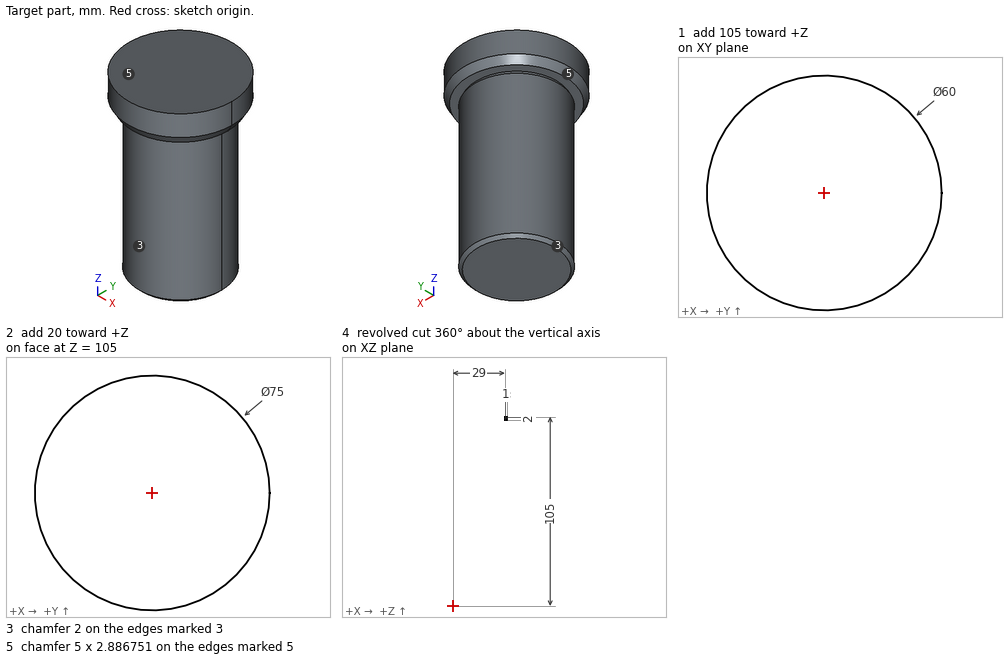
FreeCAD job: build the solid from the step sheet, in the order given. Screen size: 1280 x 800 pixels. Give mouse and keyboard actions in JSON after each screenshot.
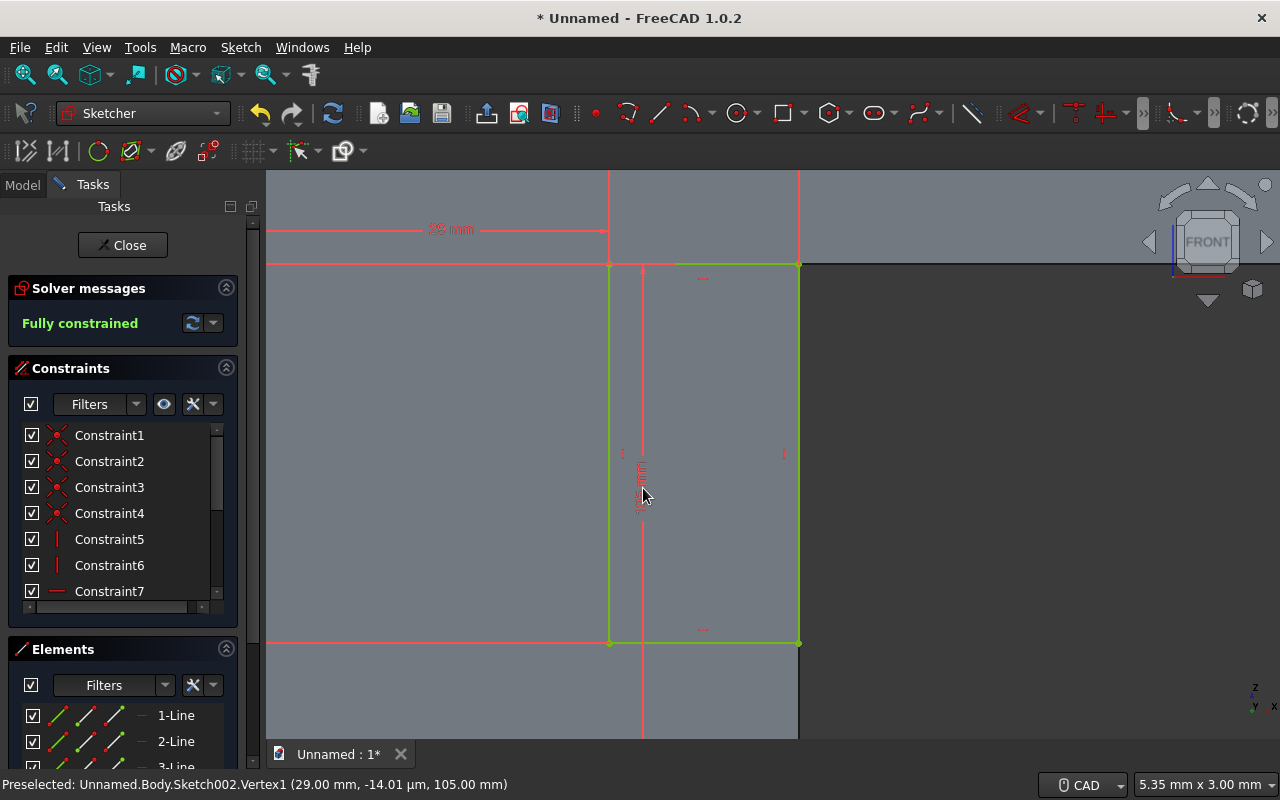
{"action": "left_click", "coordinate": [123, 245]}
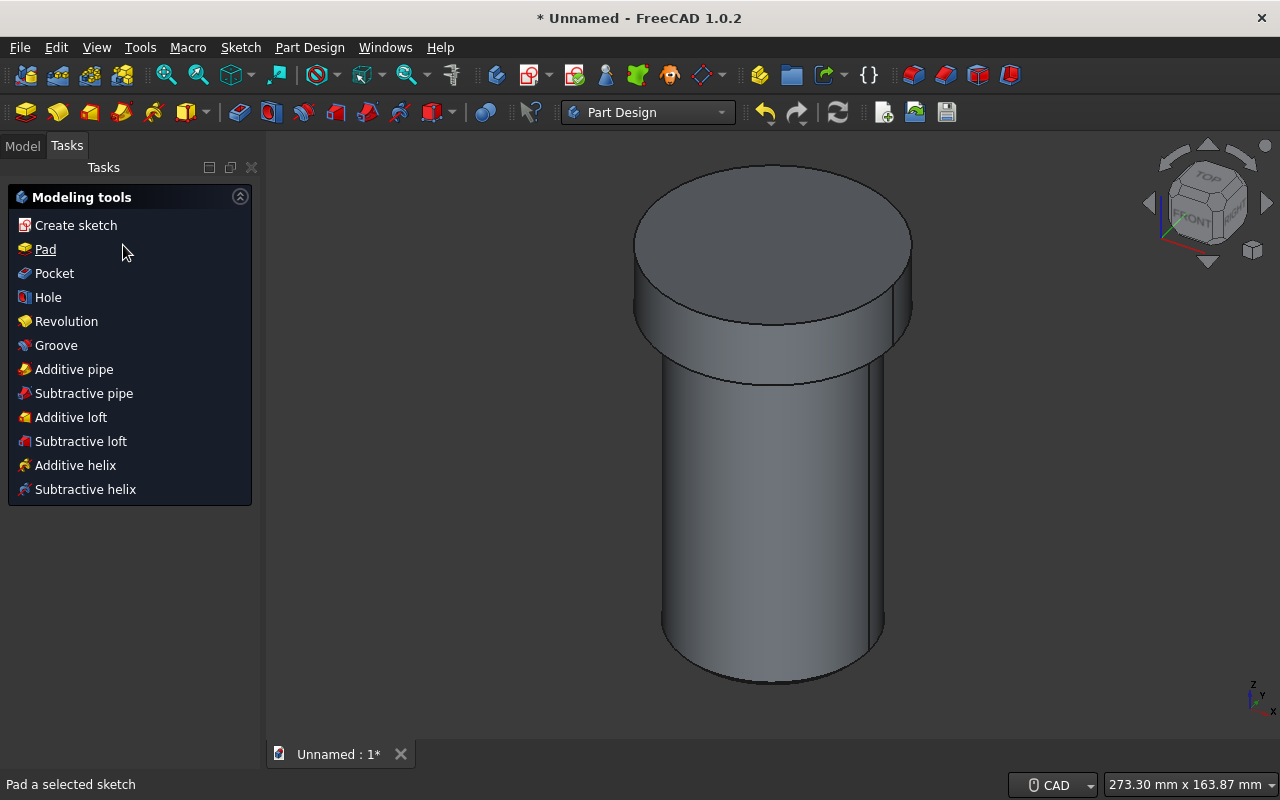
{"action": "left_click", "coordinate": [304, 112]}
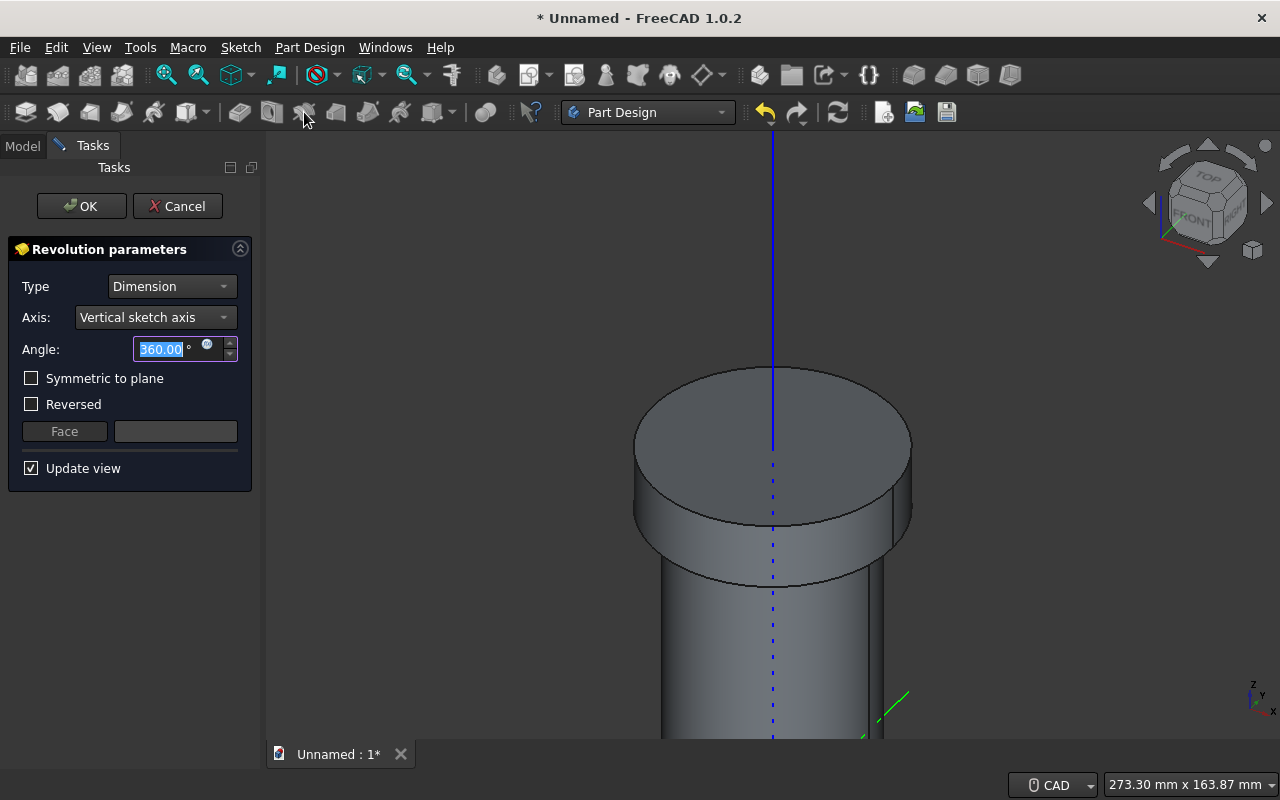
{"action": "left_click", "coordinate": [82, 206]}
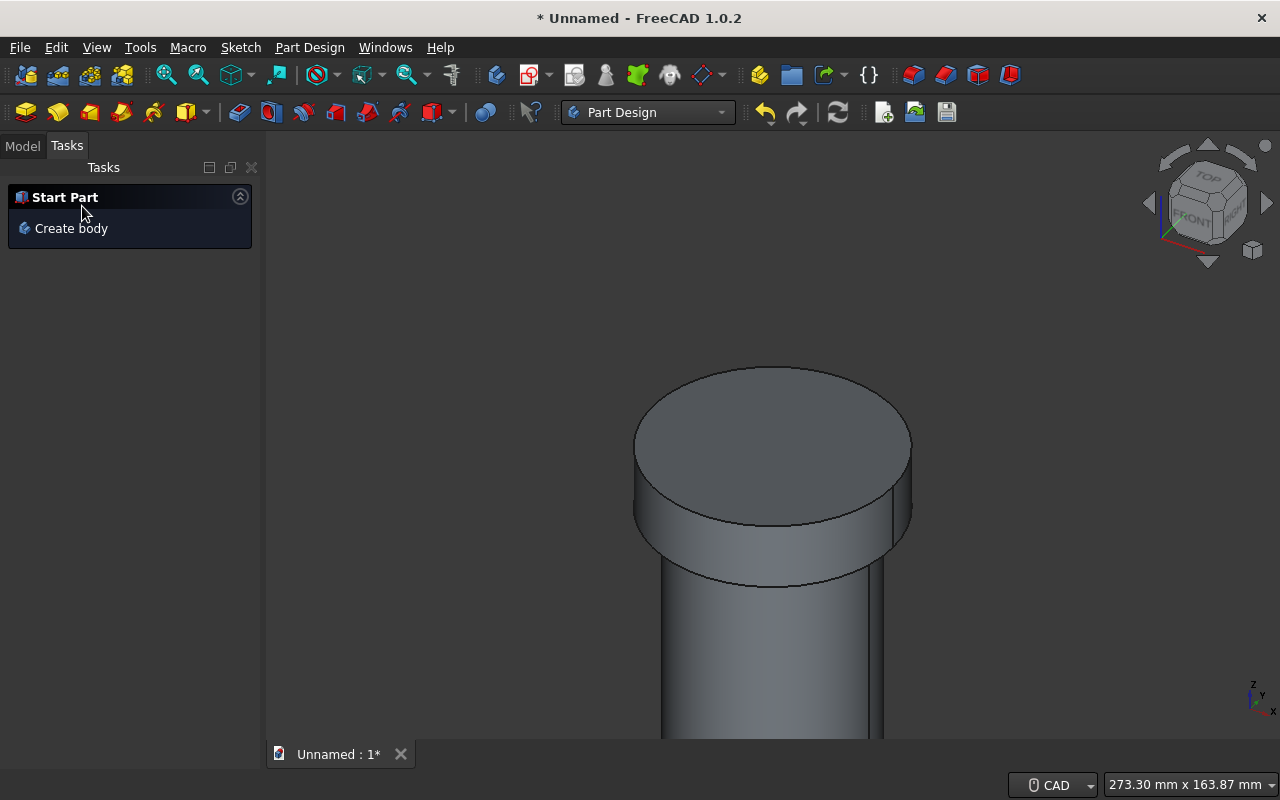
{"action": "left_click", "coordinate": [168, 76]}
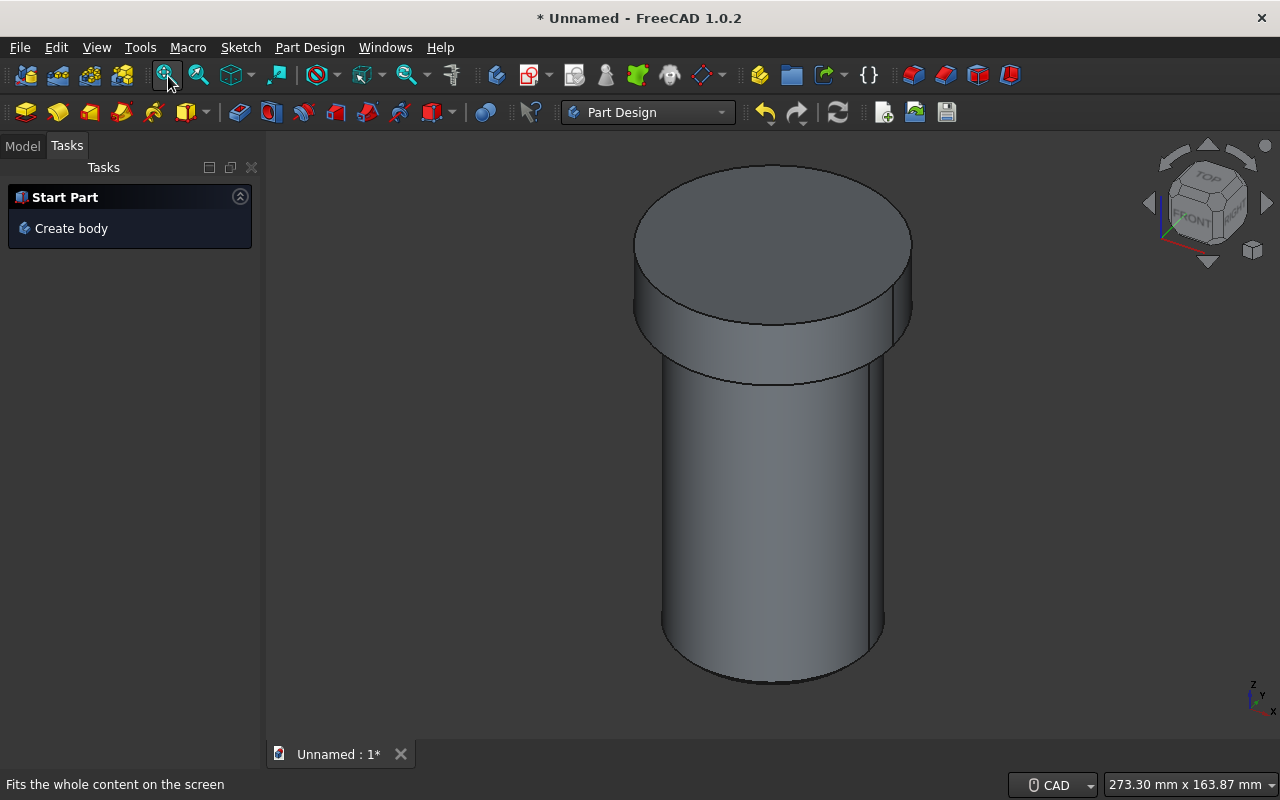
{"action": "key", "text": "0"}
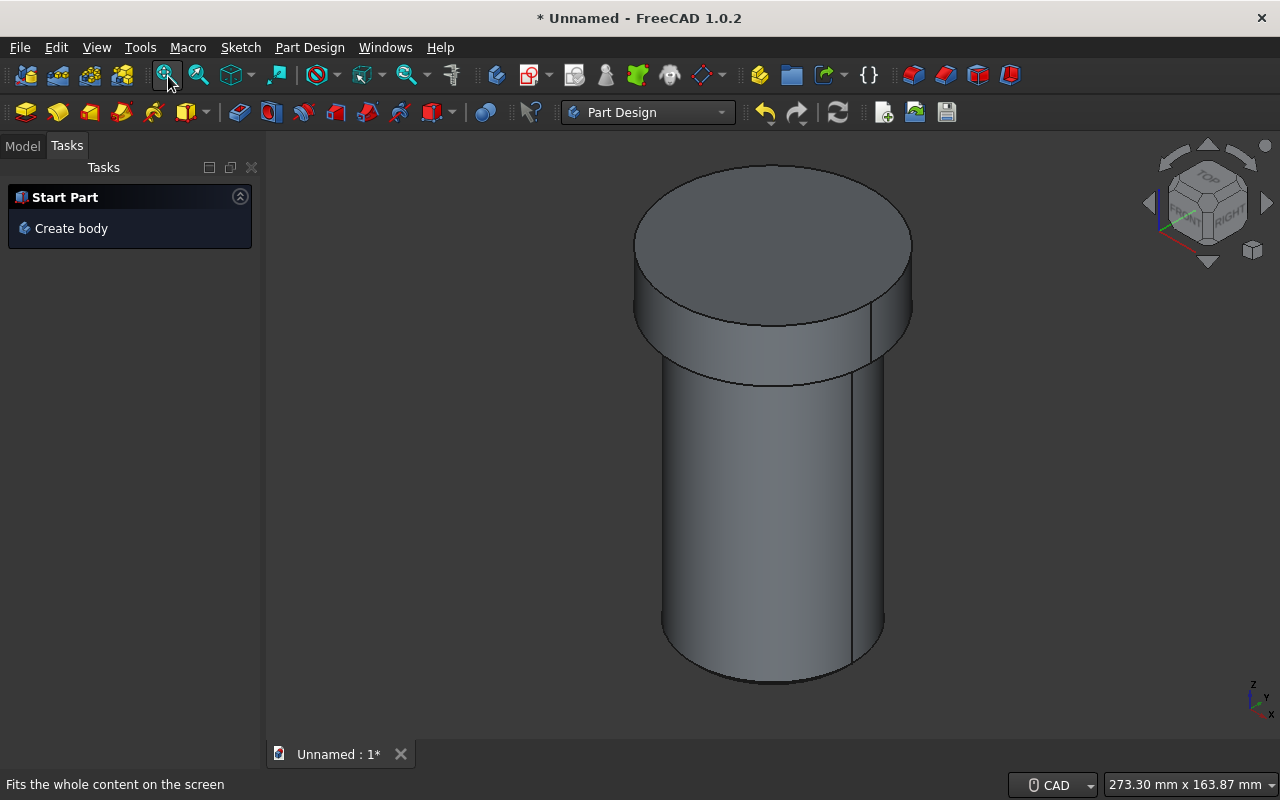
{"action": "key", "text": "2"}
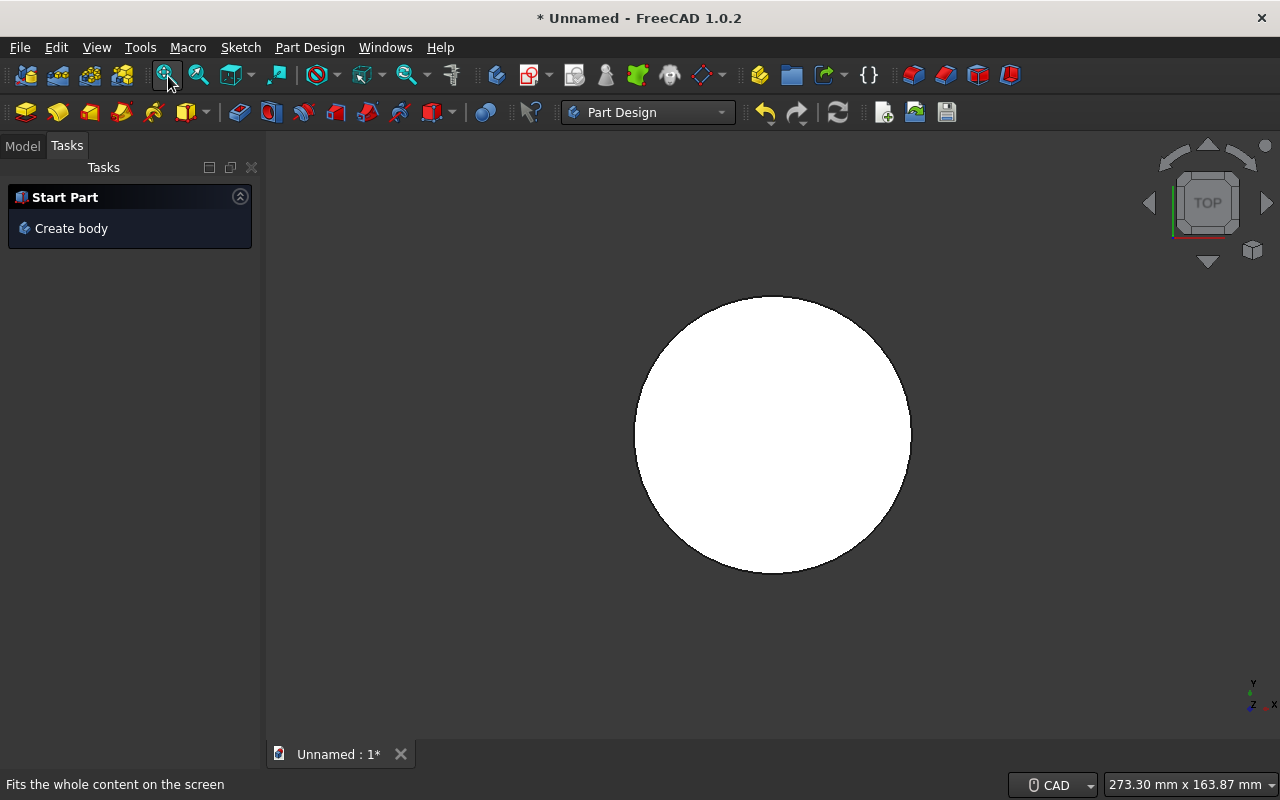
{"action": "key", "text": "1"}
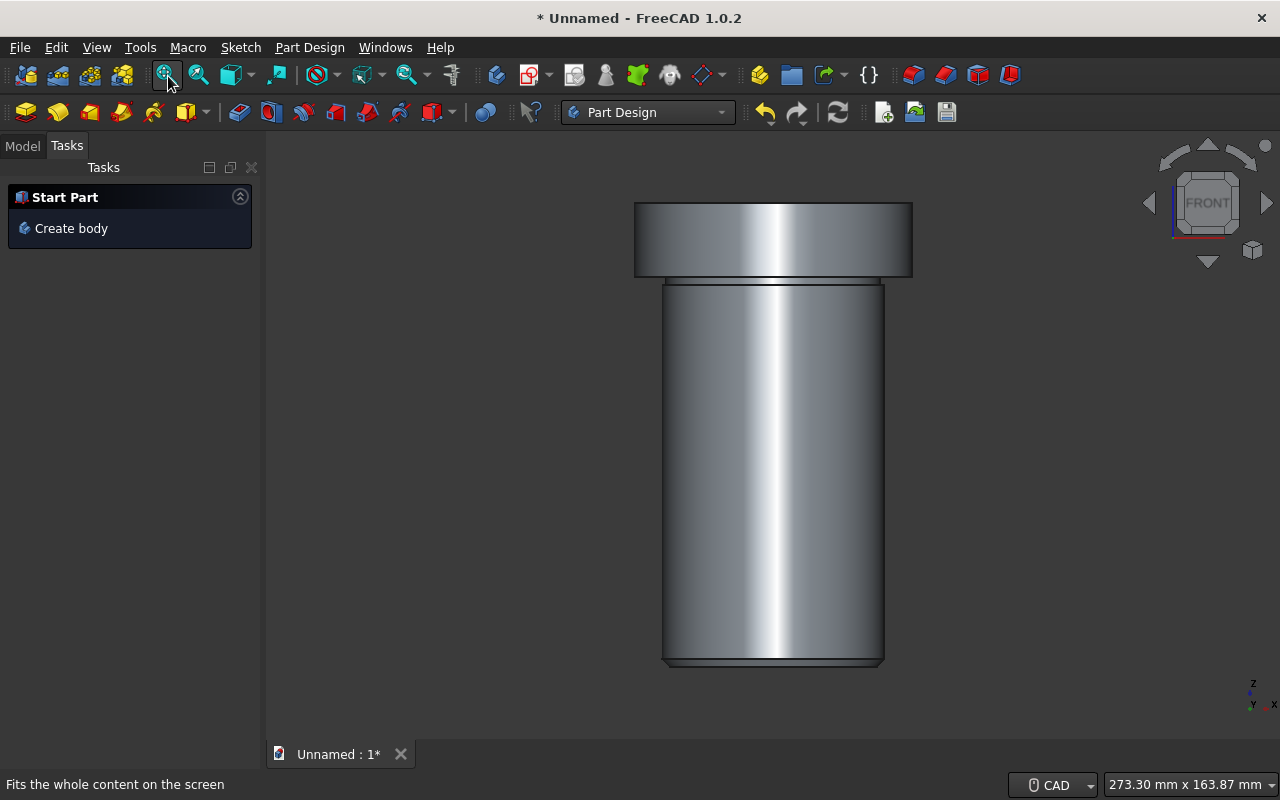
{"action": "left_click", "coordinate": [660, 276]}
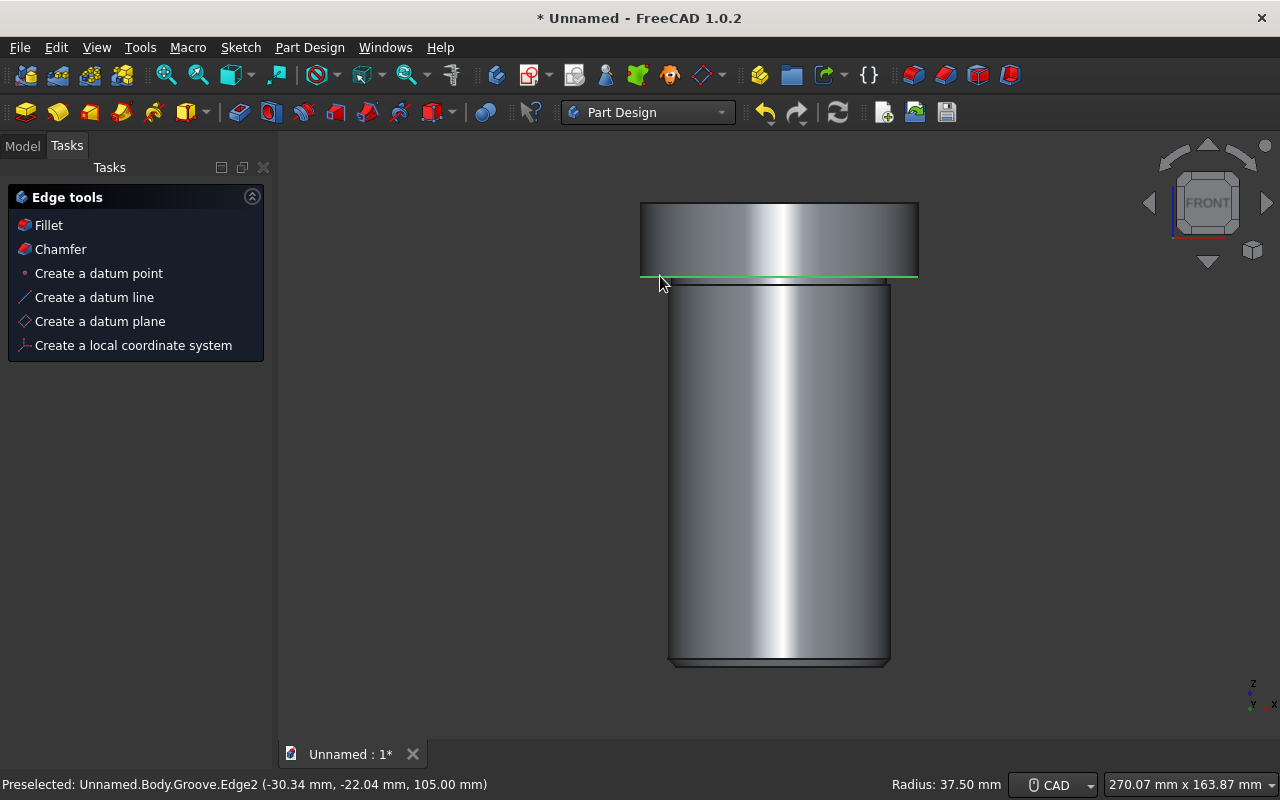
{"action": "left_click", "coordinate": [946, 76]}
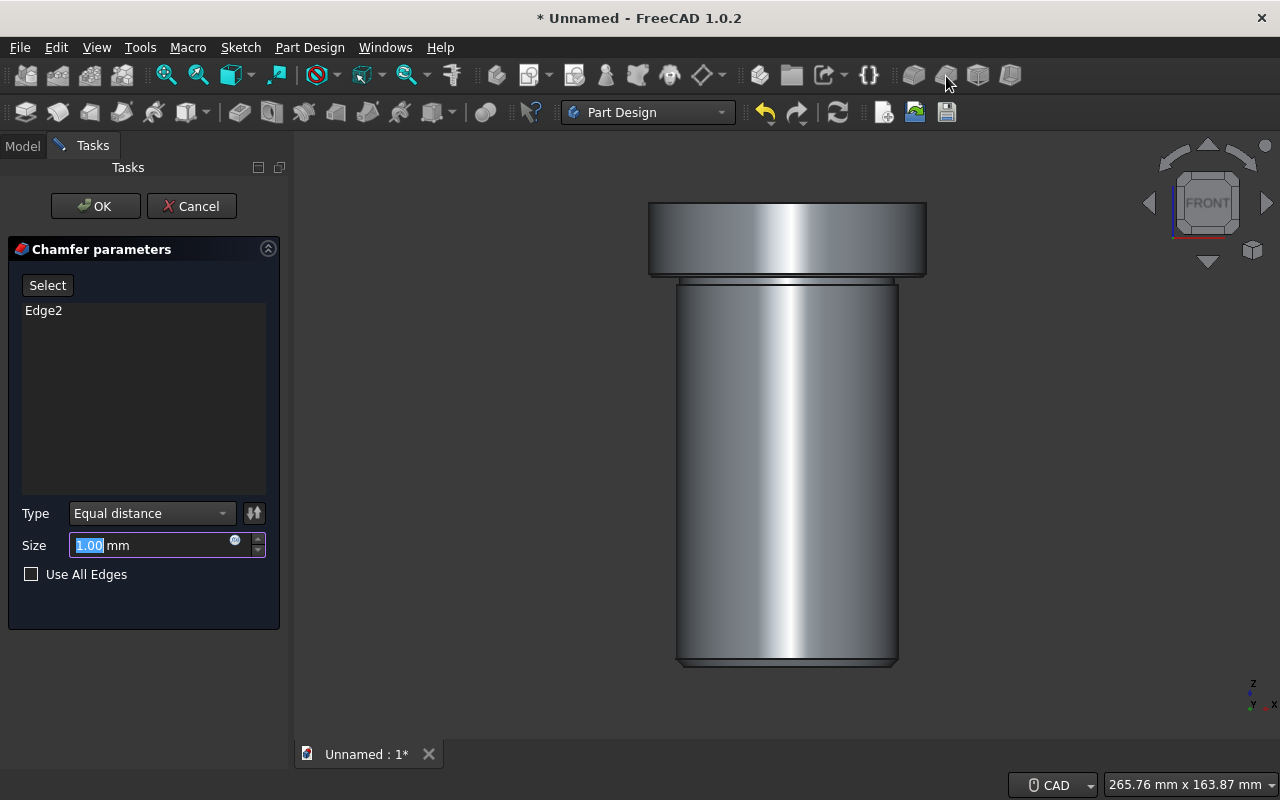
{"action": "type", "text": "5"}
{"action": "key", "text": "Tab"}